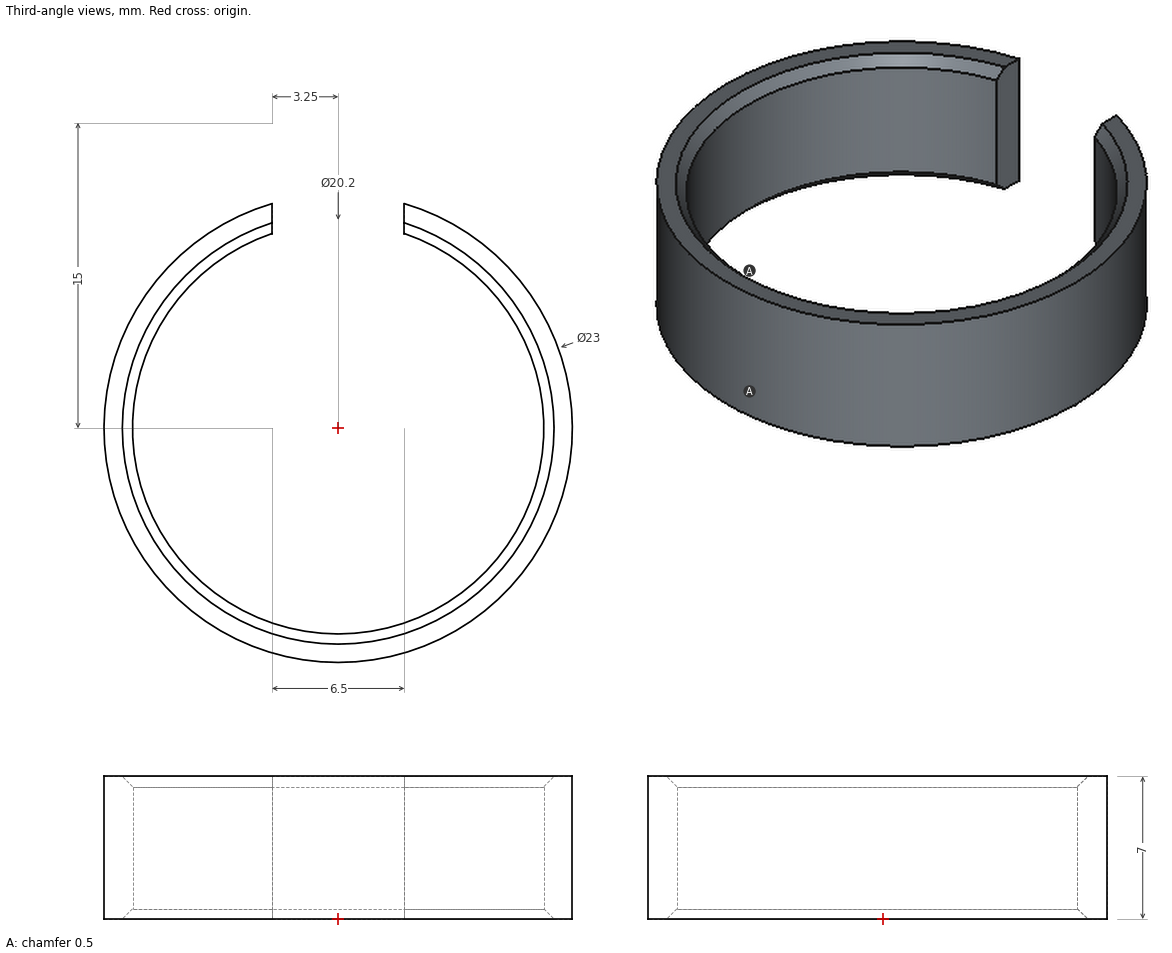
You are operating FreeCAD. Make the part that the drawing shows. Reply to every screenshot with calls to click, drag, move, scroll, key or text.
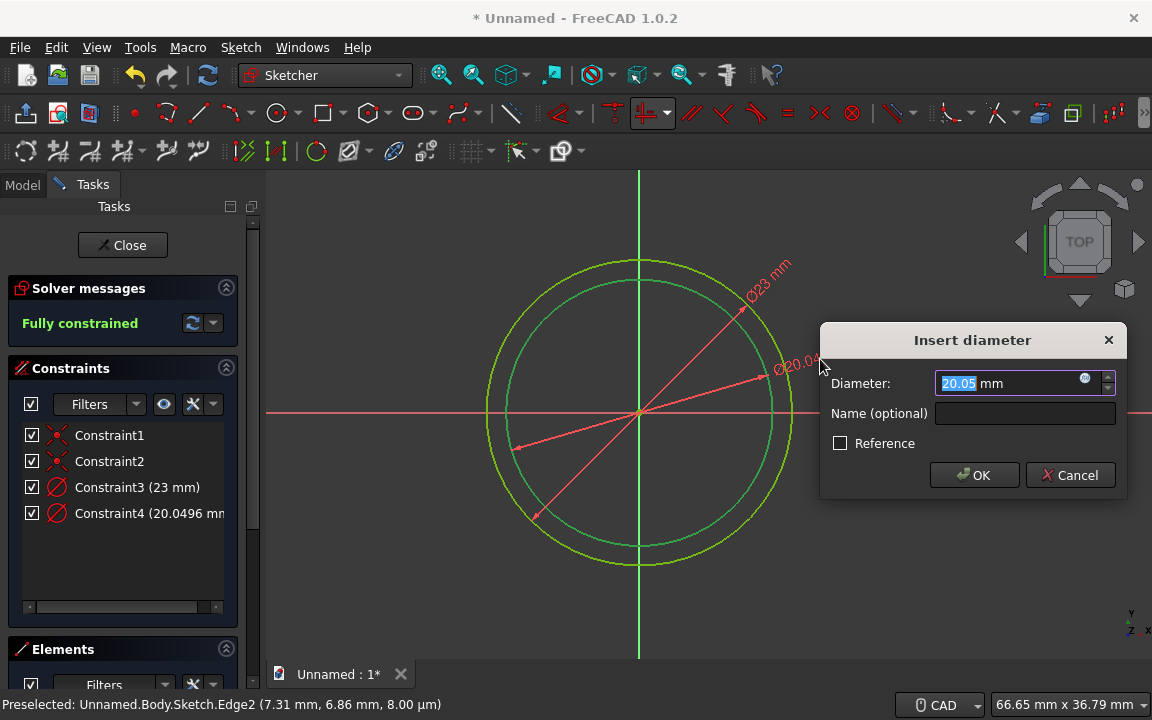
text(20.2)
key(Return)
key(Escape)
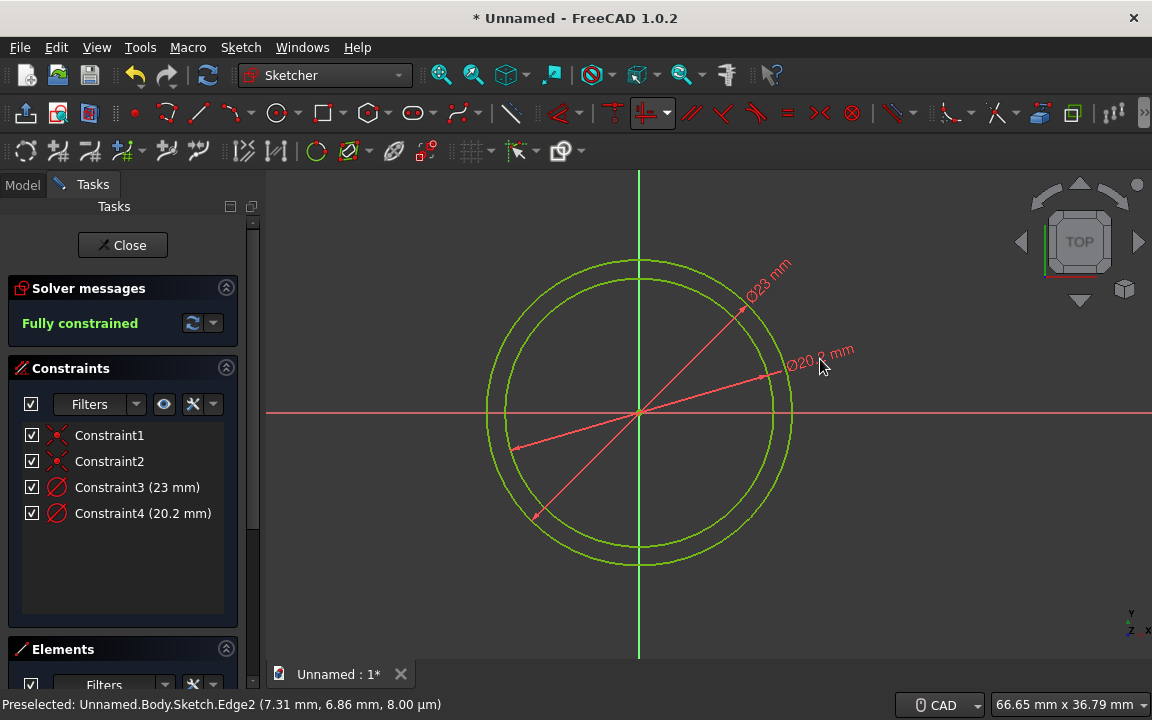
click(123, 245)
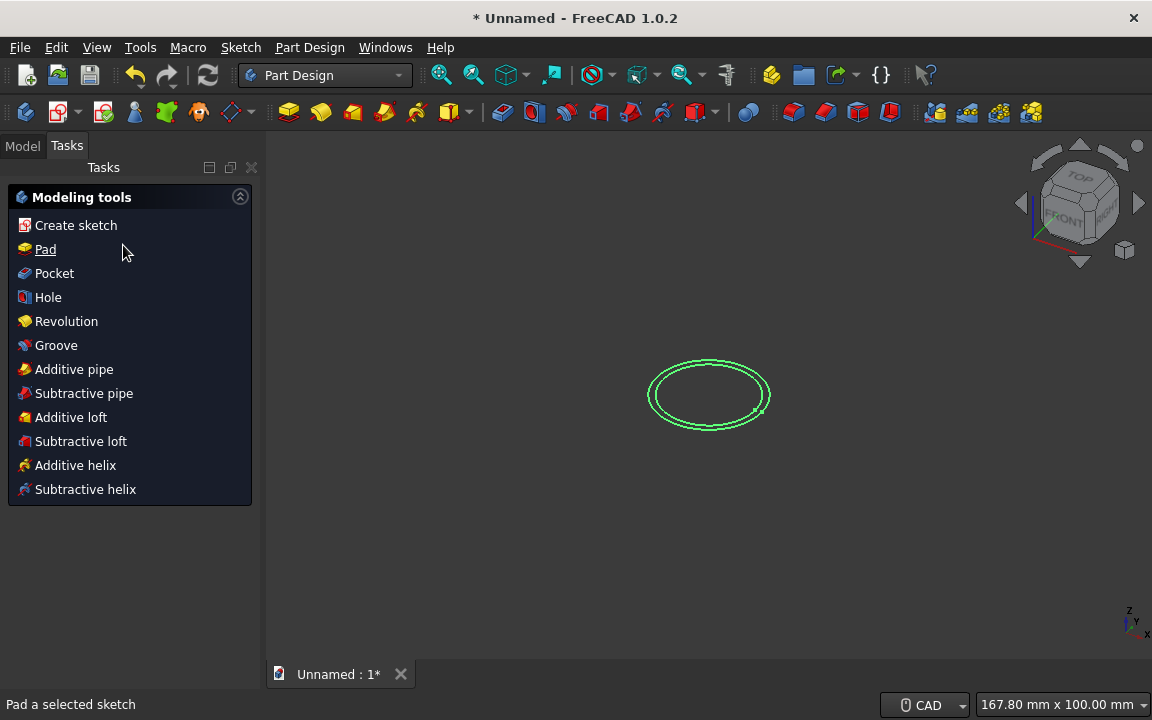
click(290, 112)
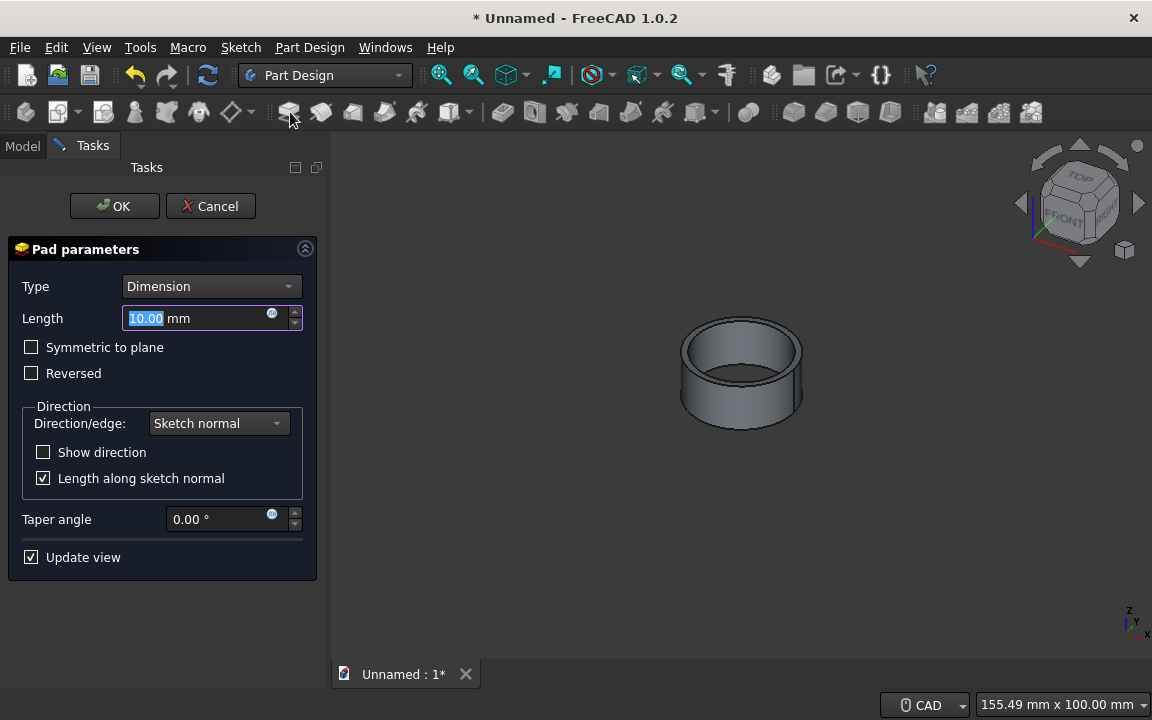
text(7)
key(Tab)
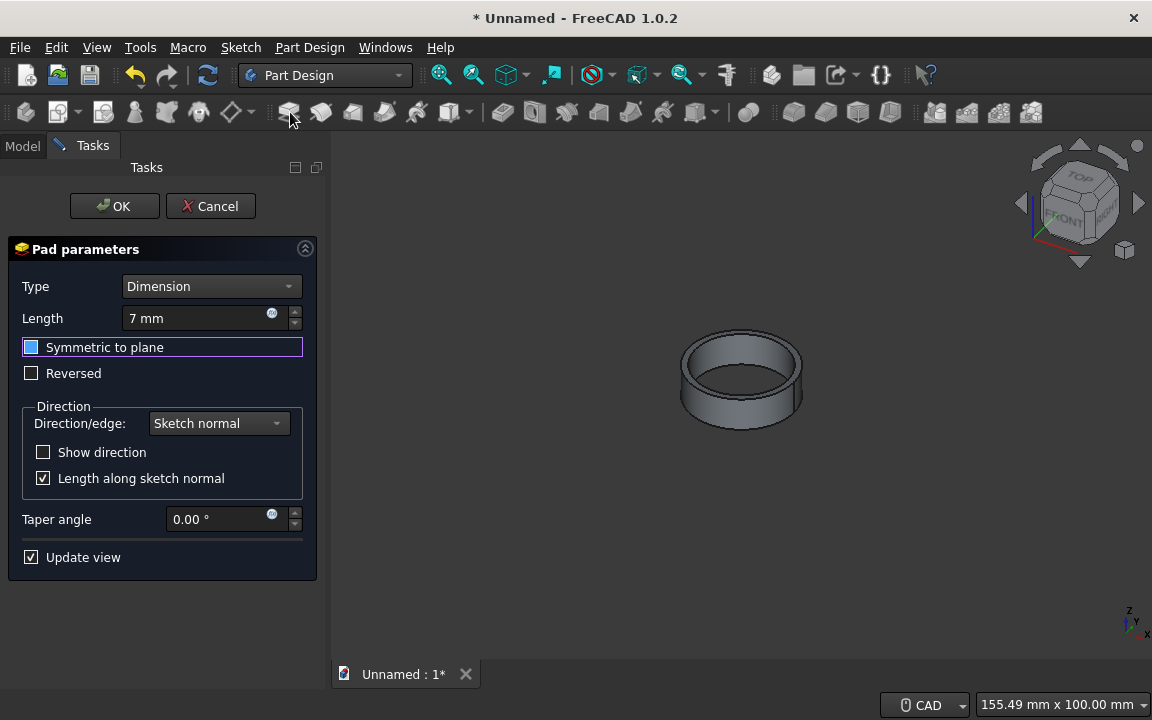
click(115, 206)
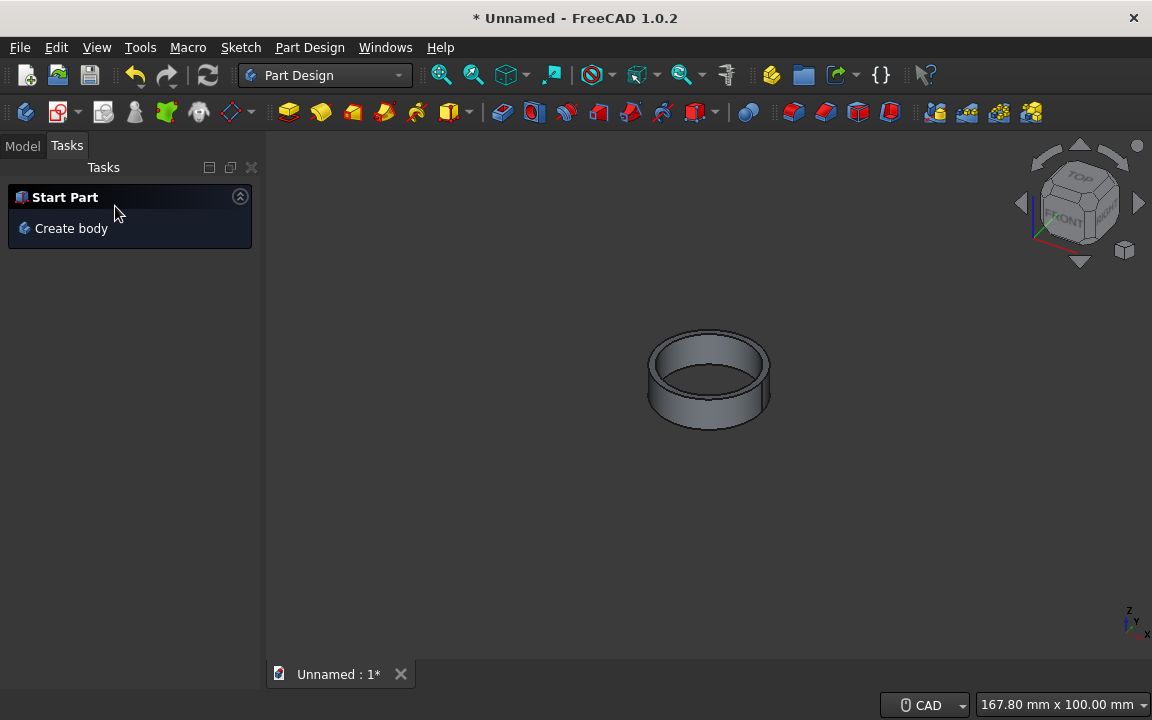
click(442, 76)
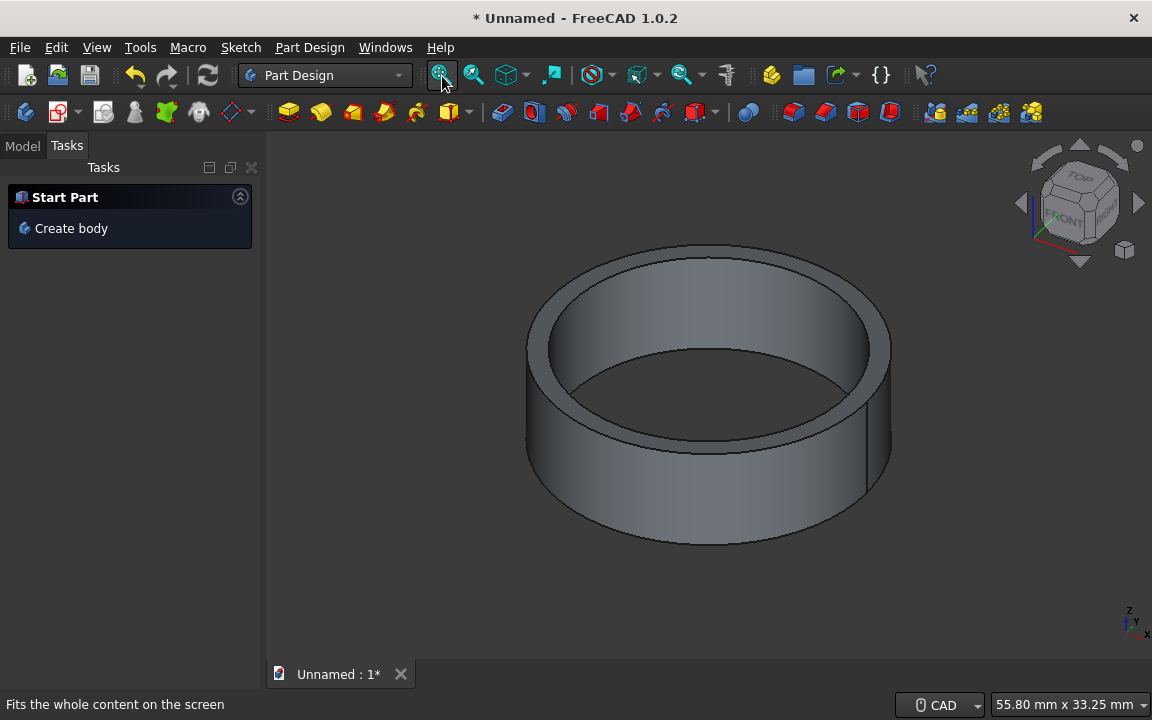
scroll(599, 278, up, 5)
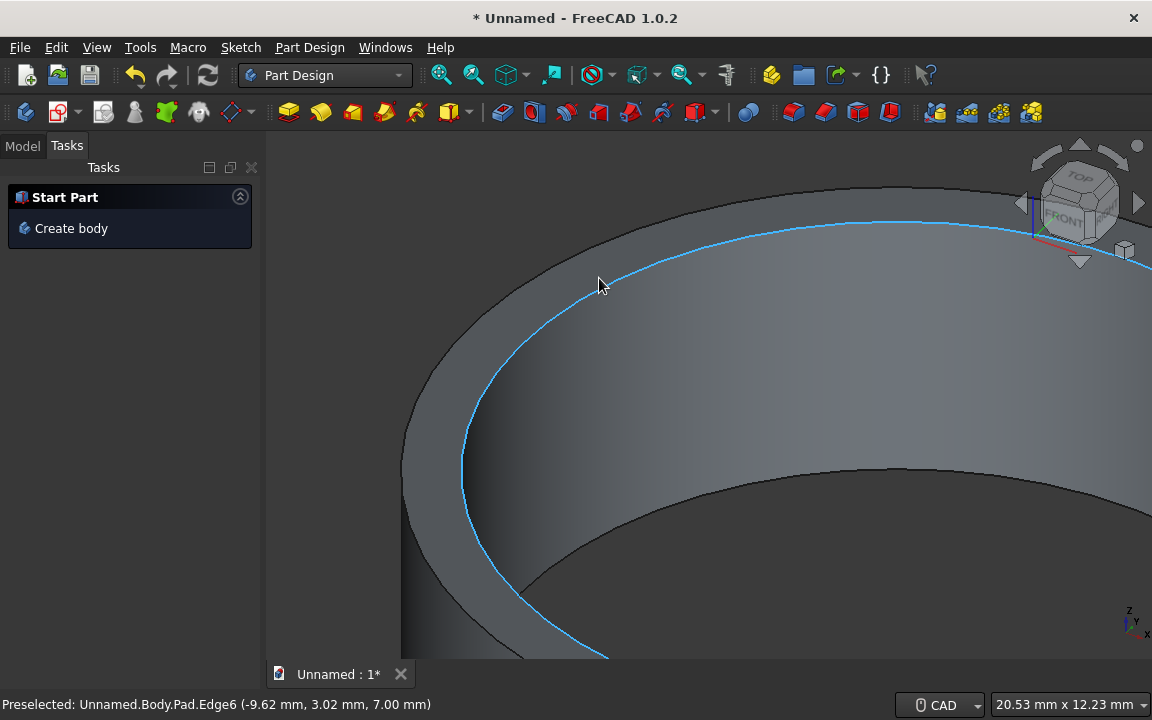
click(458, 419)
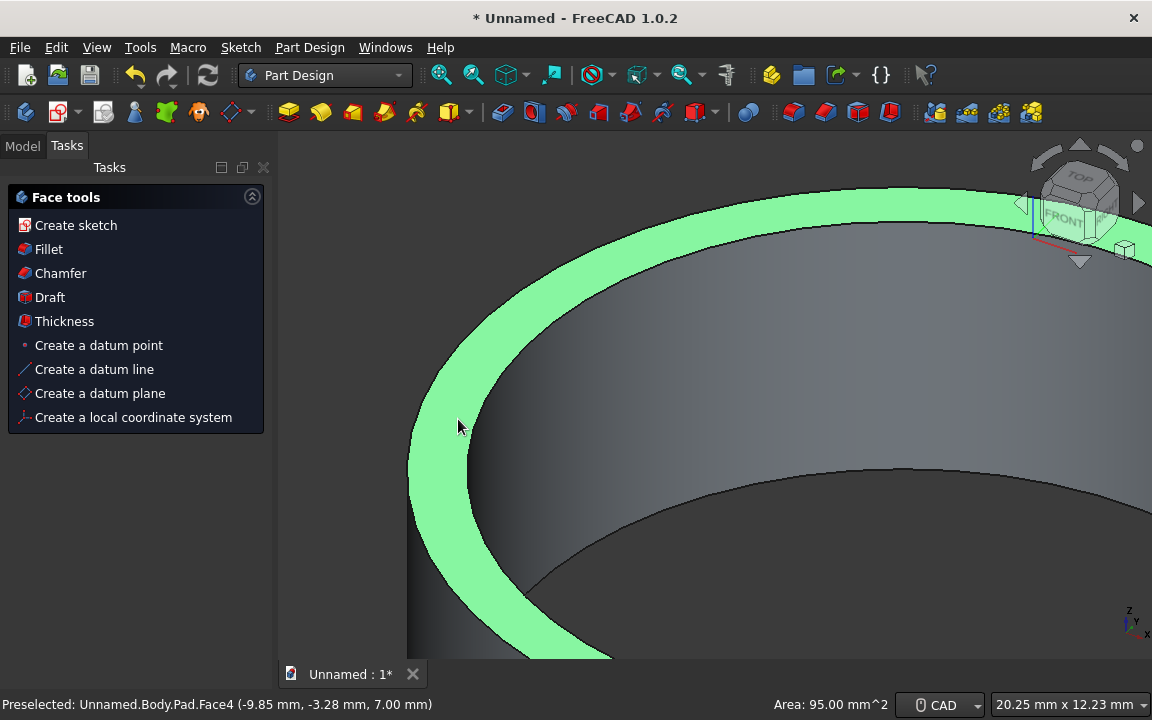
click(58, 112)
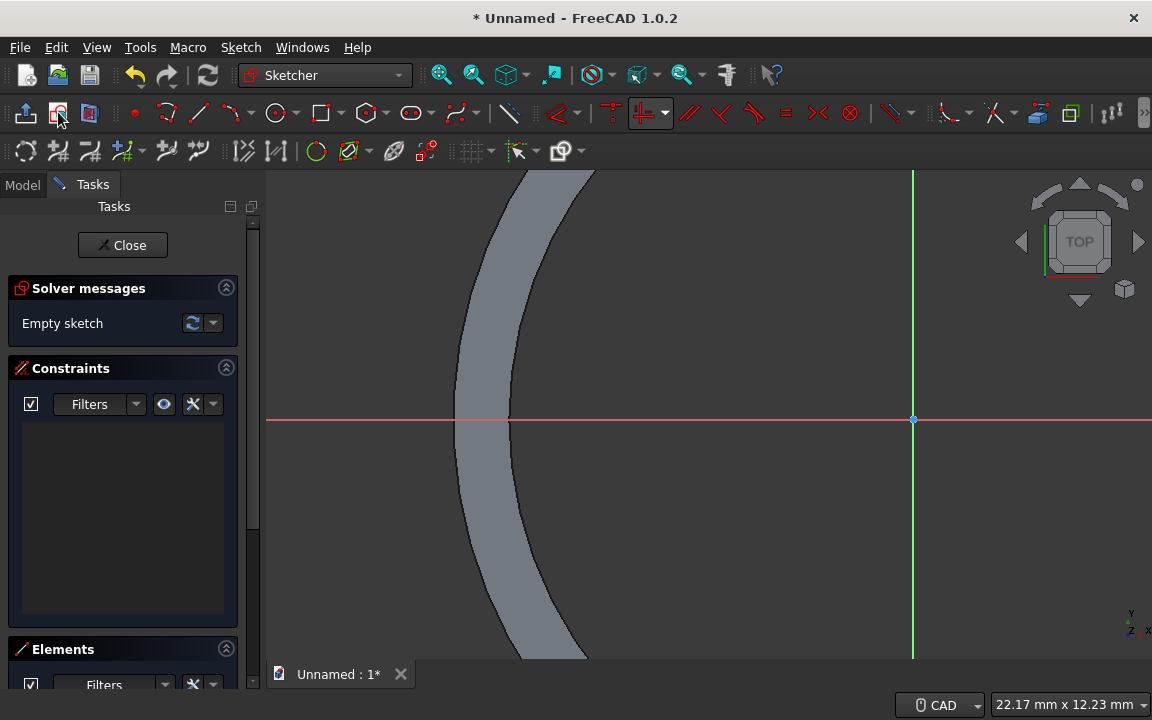
scroll(418, 631, down, 4)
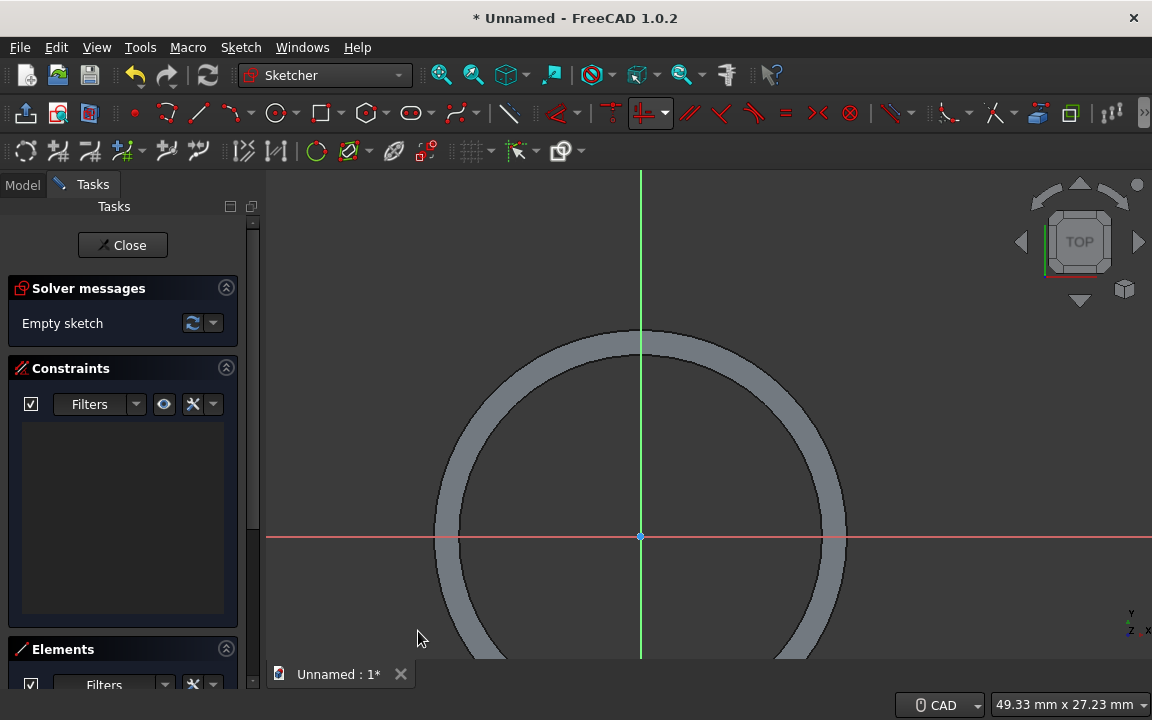
click(322, 114)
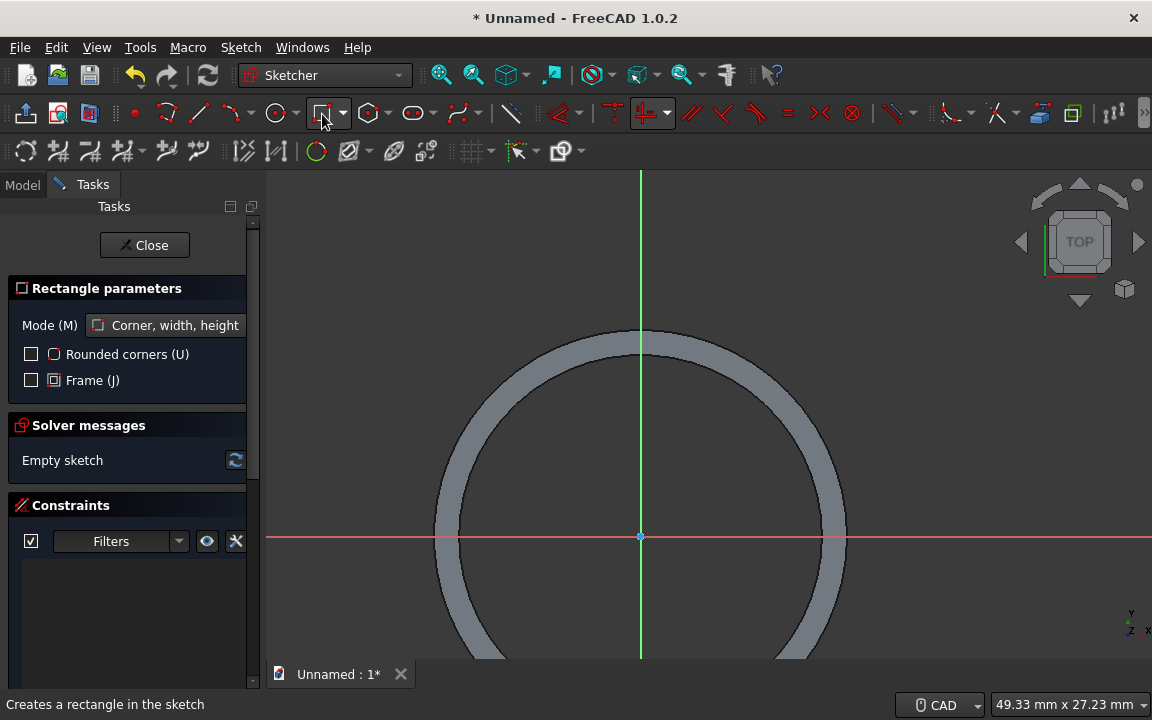
click(582, 267)
click(699, 537)
key(Escape)